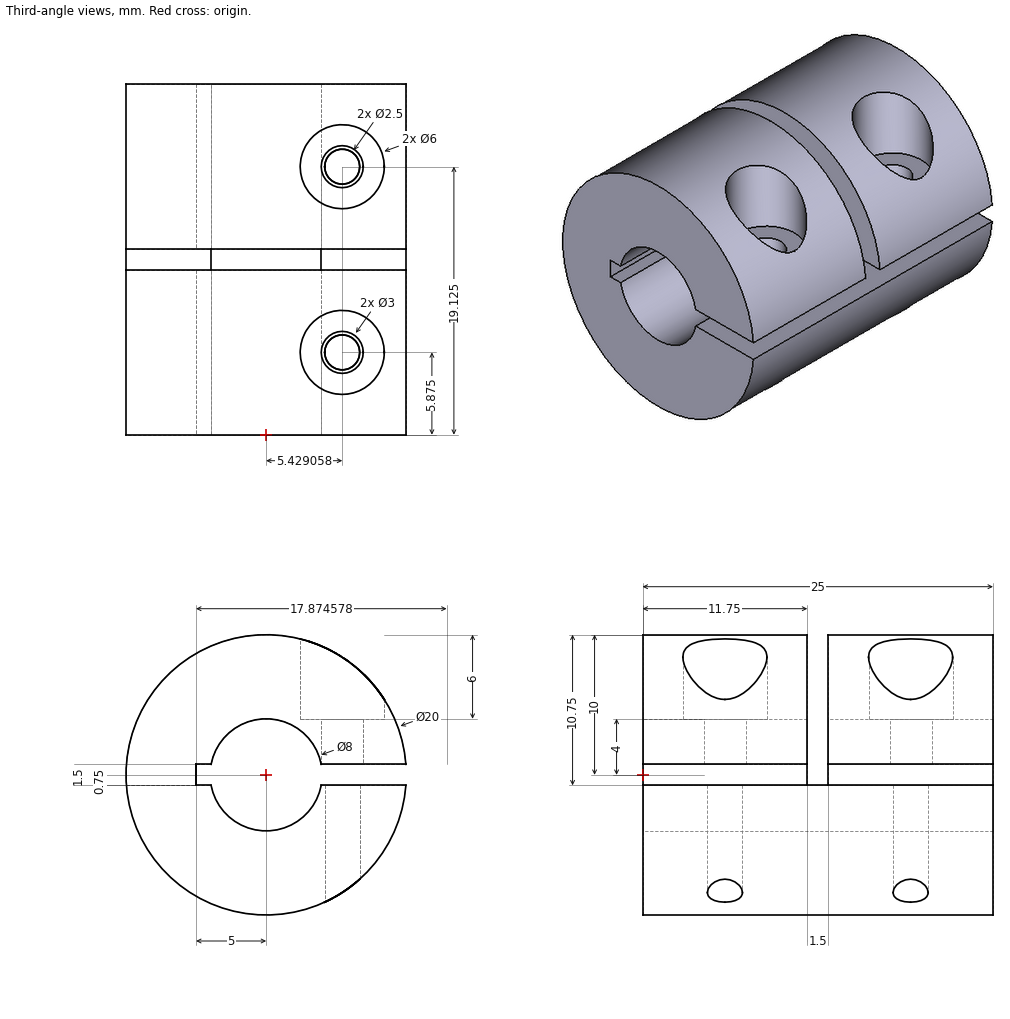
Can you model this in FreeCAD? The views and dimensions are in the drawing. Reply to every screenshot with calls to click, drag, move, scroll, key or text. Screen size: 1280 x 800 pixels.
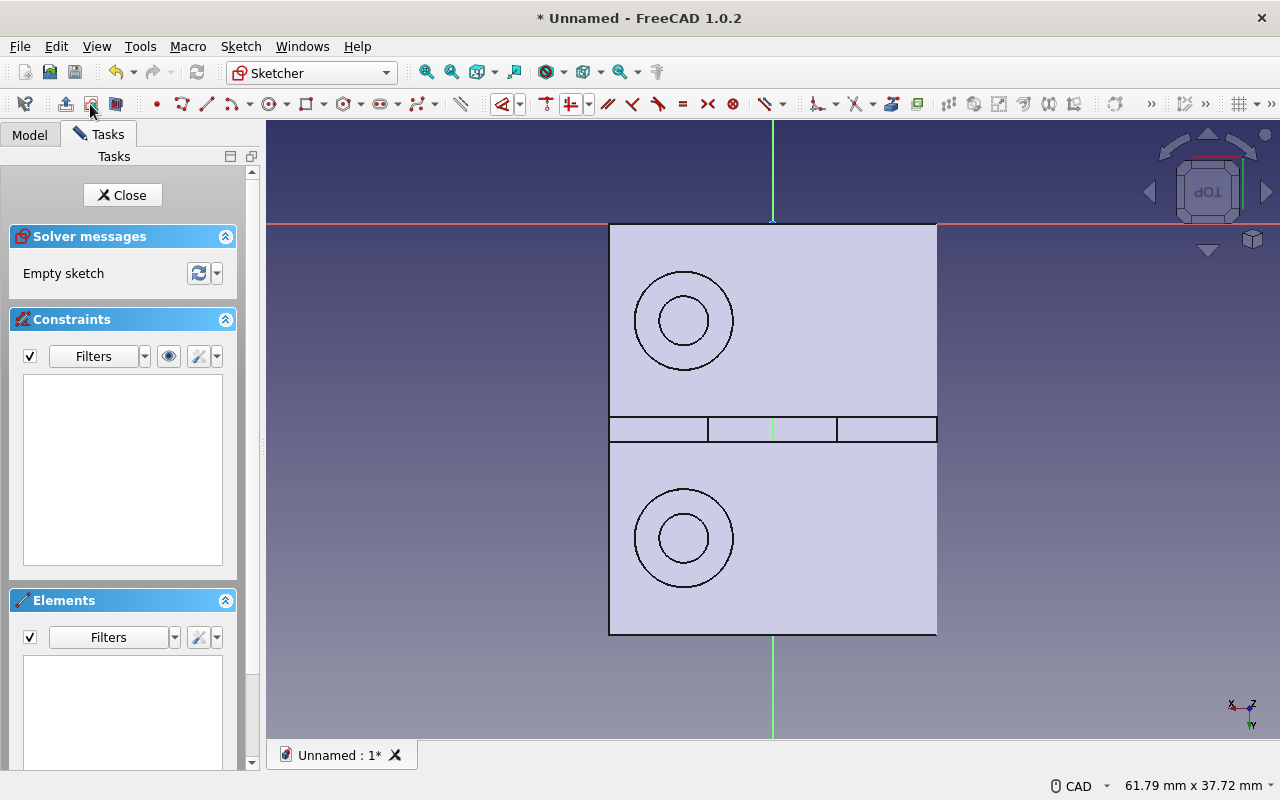
click(116, 104)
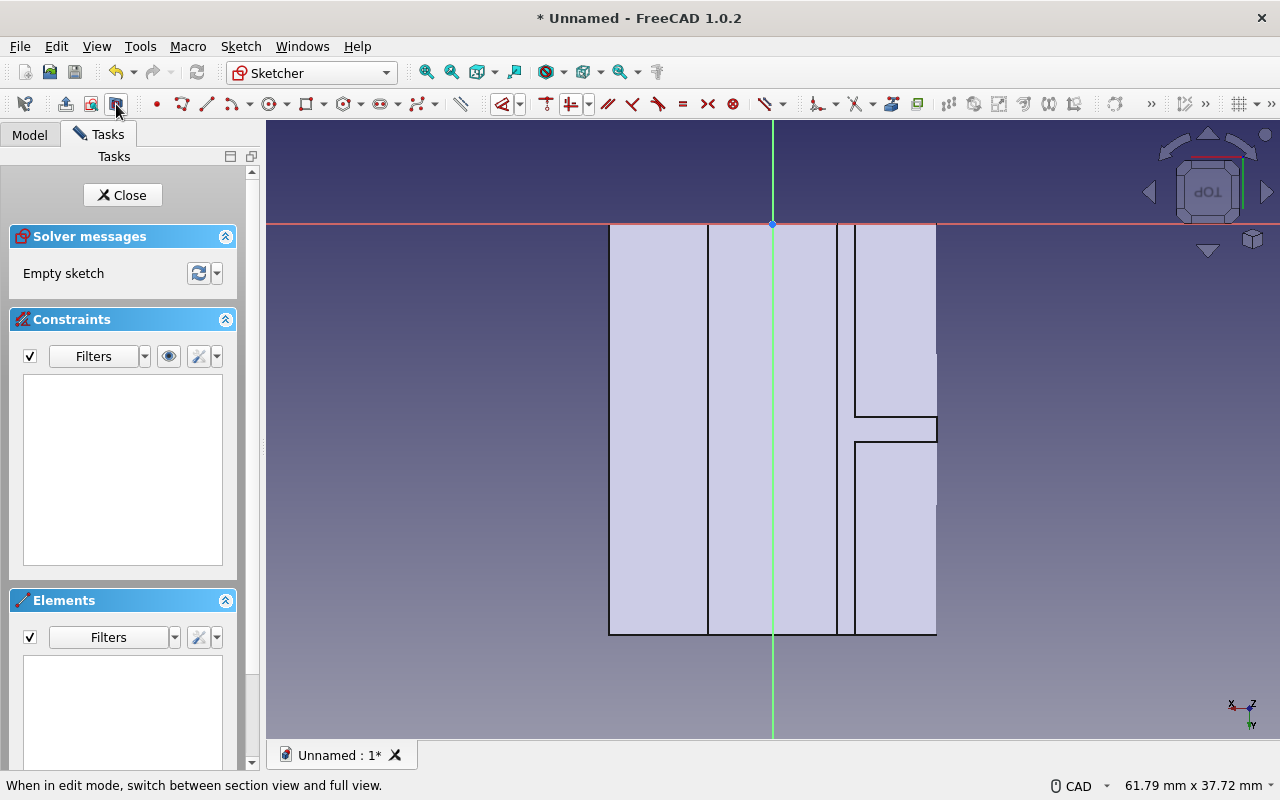
click(268, 104)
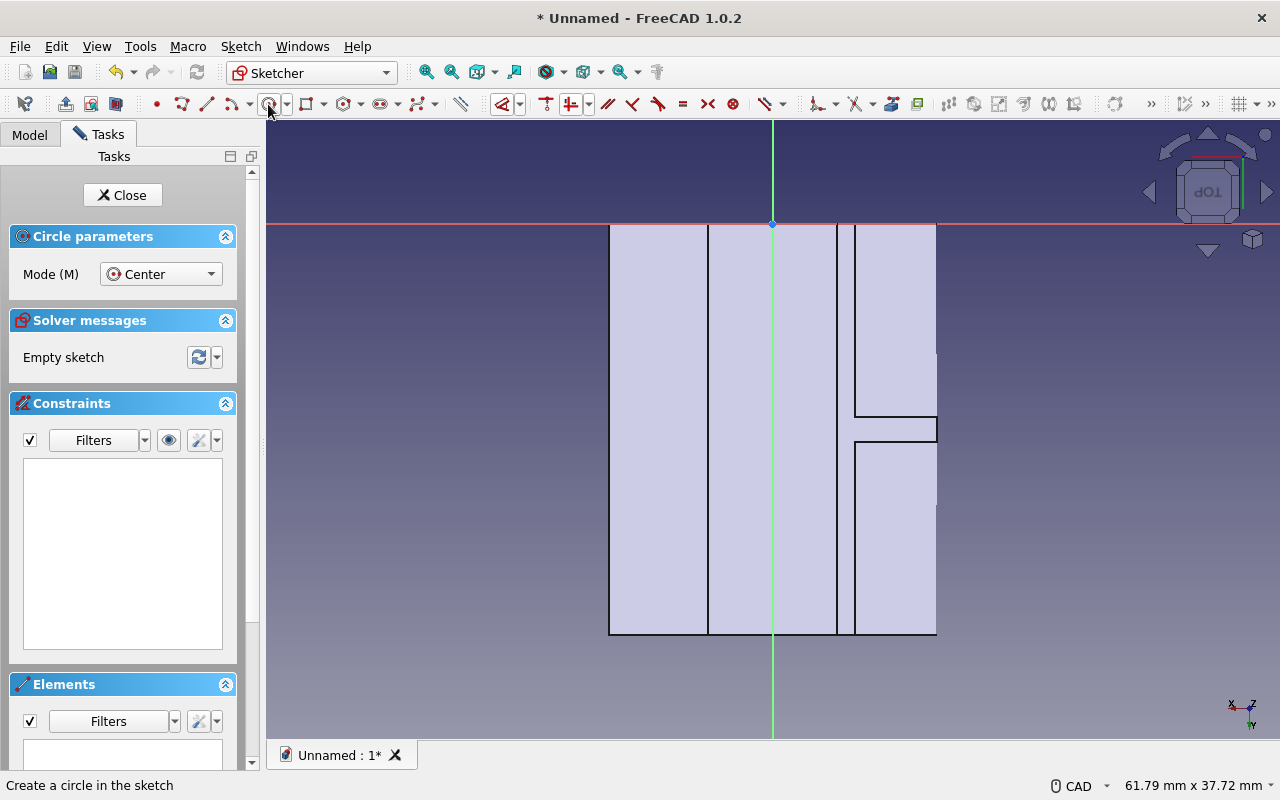
click(684, 538)
click(698, 524)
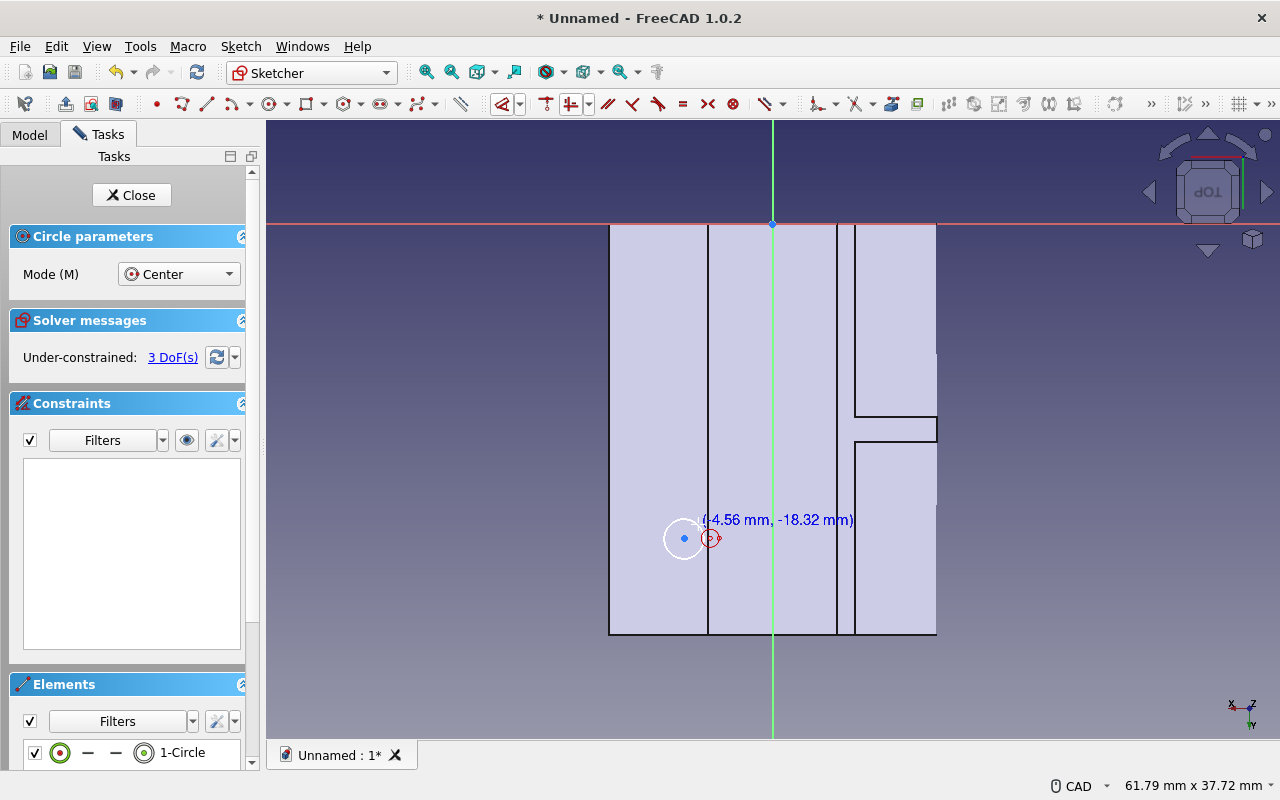
click(684, 321)
click(698, 306)
key(Escape)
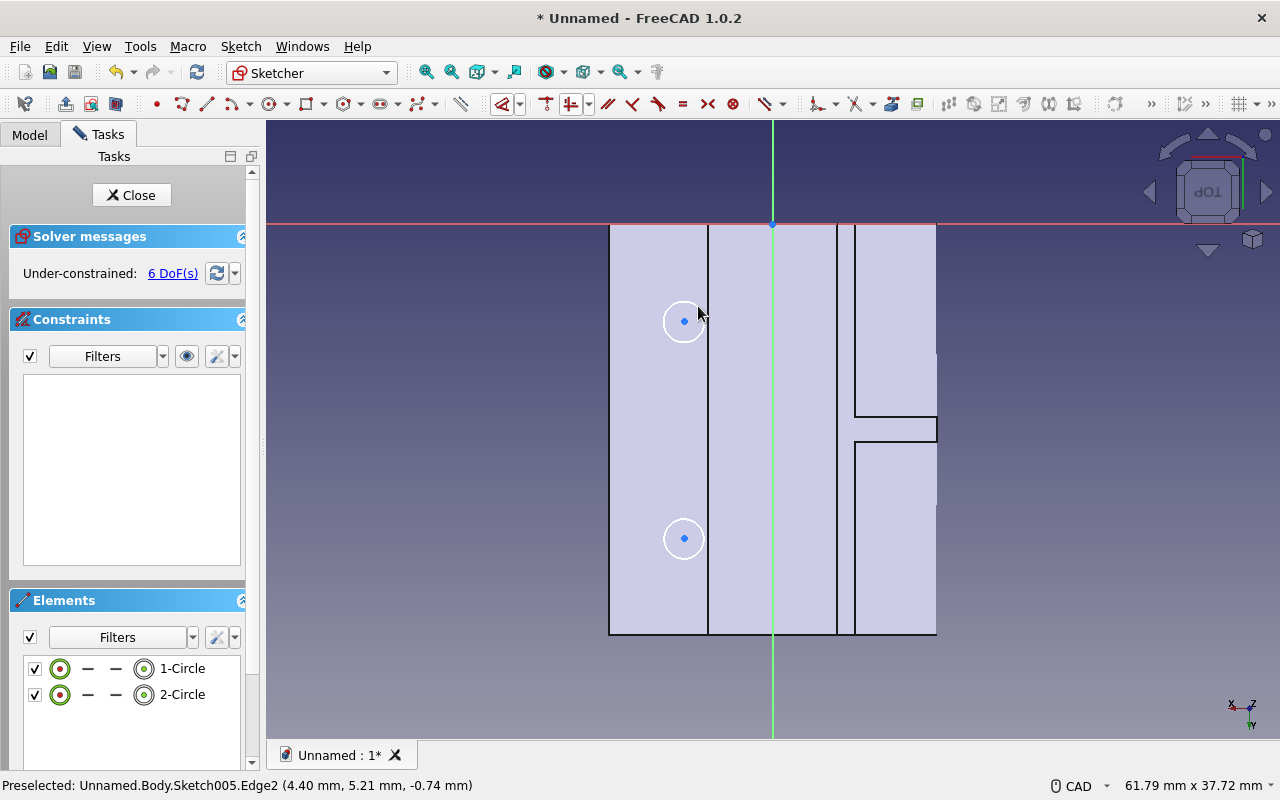
click(698, 525)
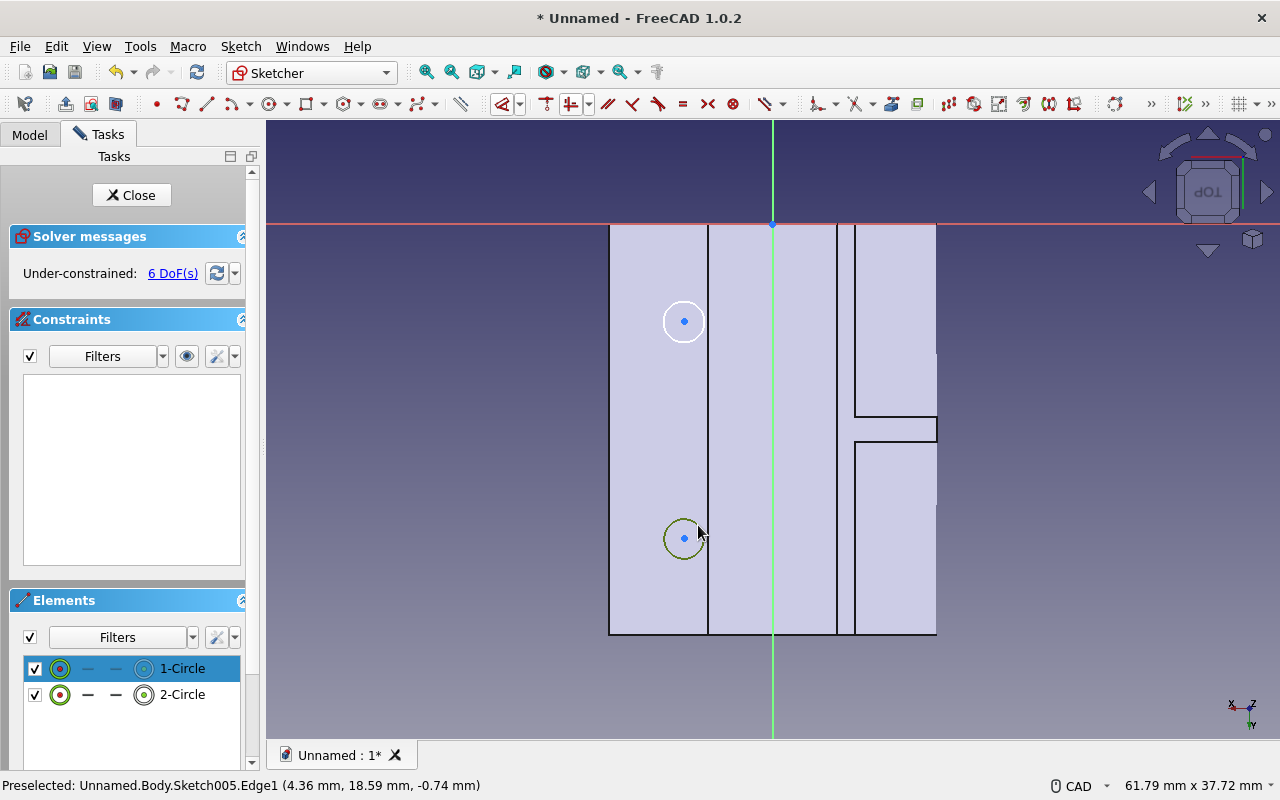
click(698, 307)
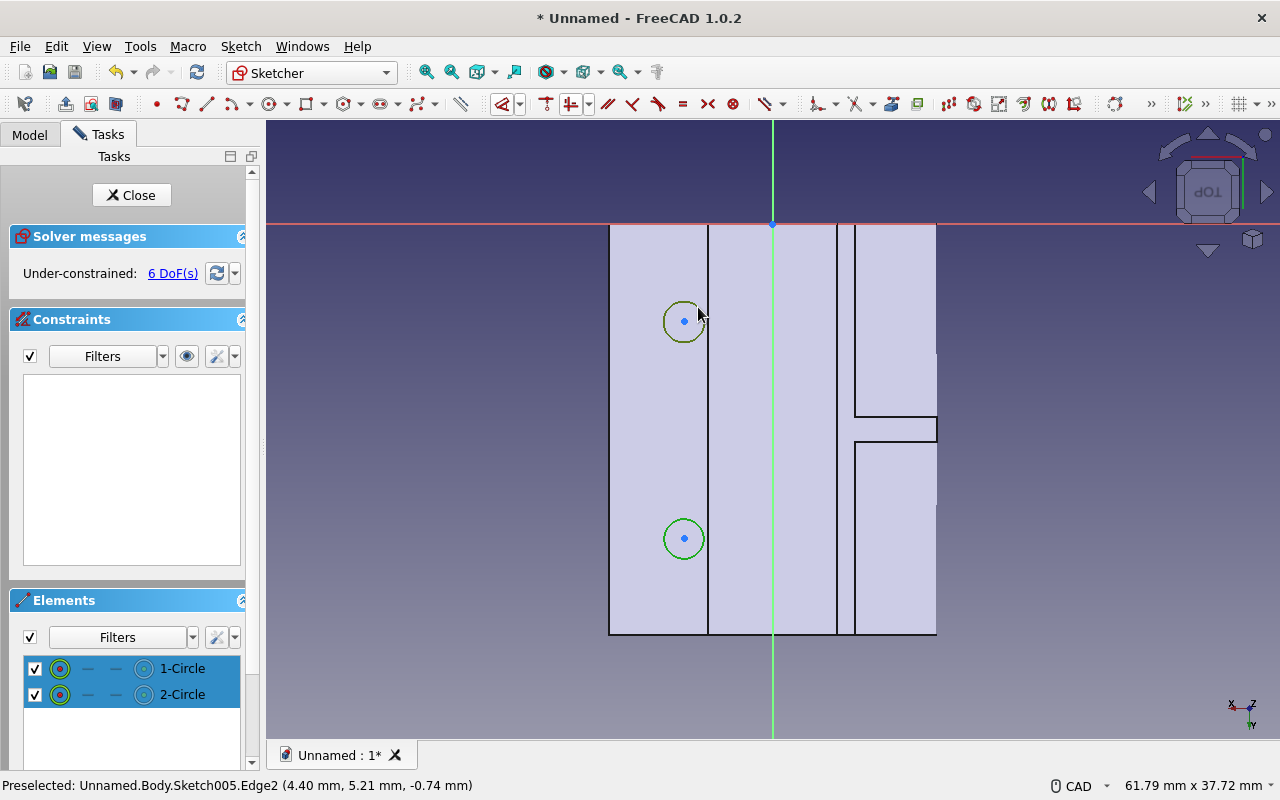
click(683, 104)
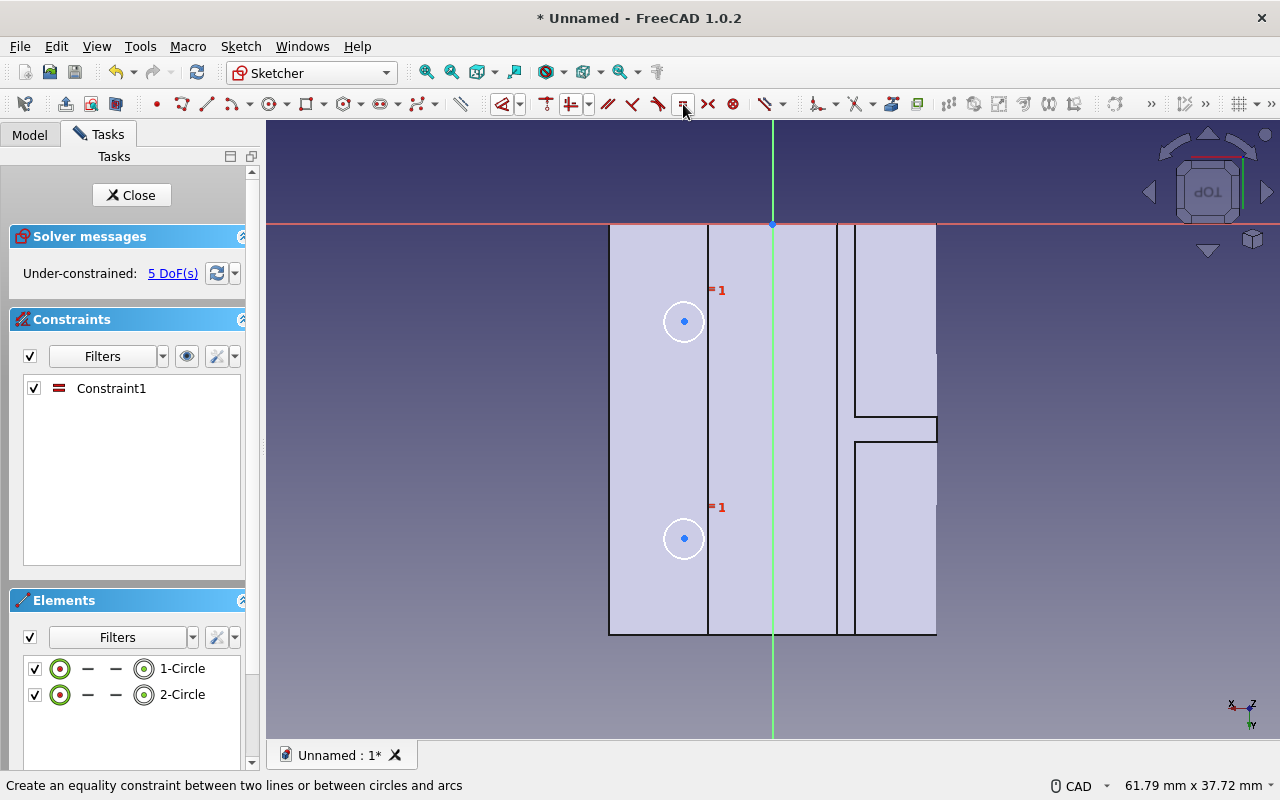
click(684, 539)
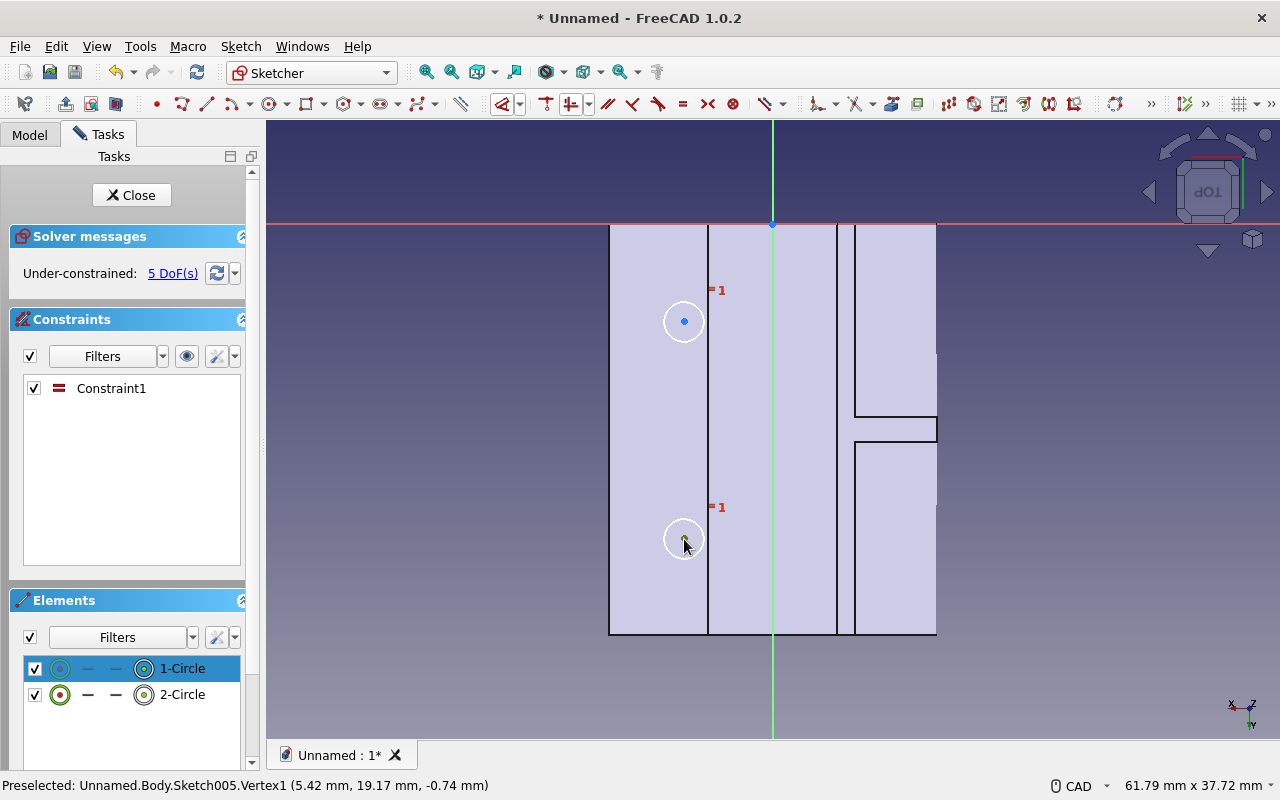
click(684, 322)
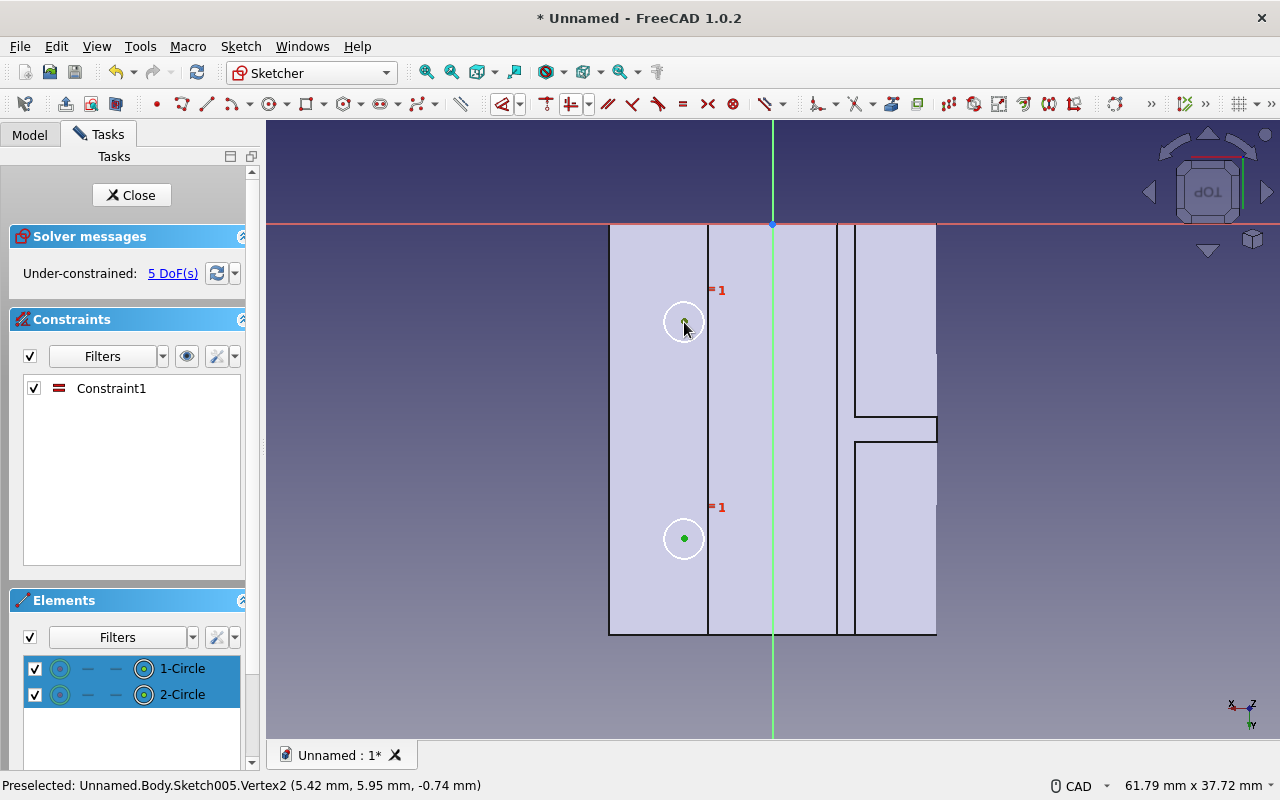
click(588, 104)